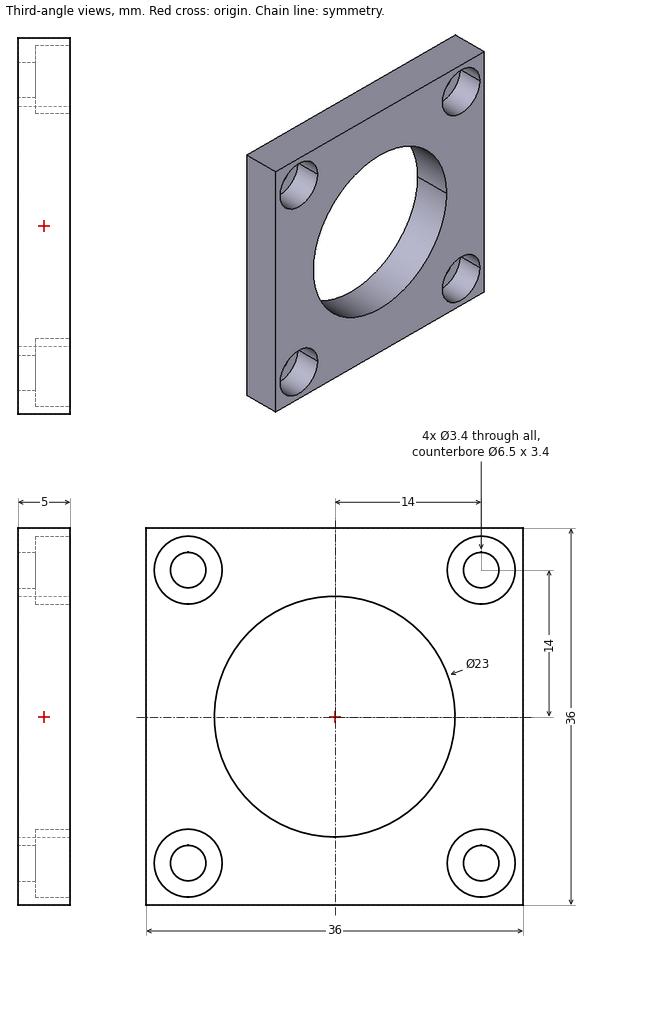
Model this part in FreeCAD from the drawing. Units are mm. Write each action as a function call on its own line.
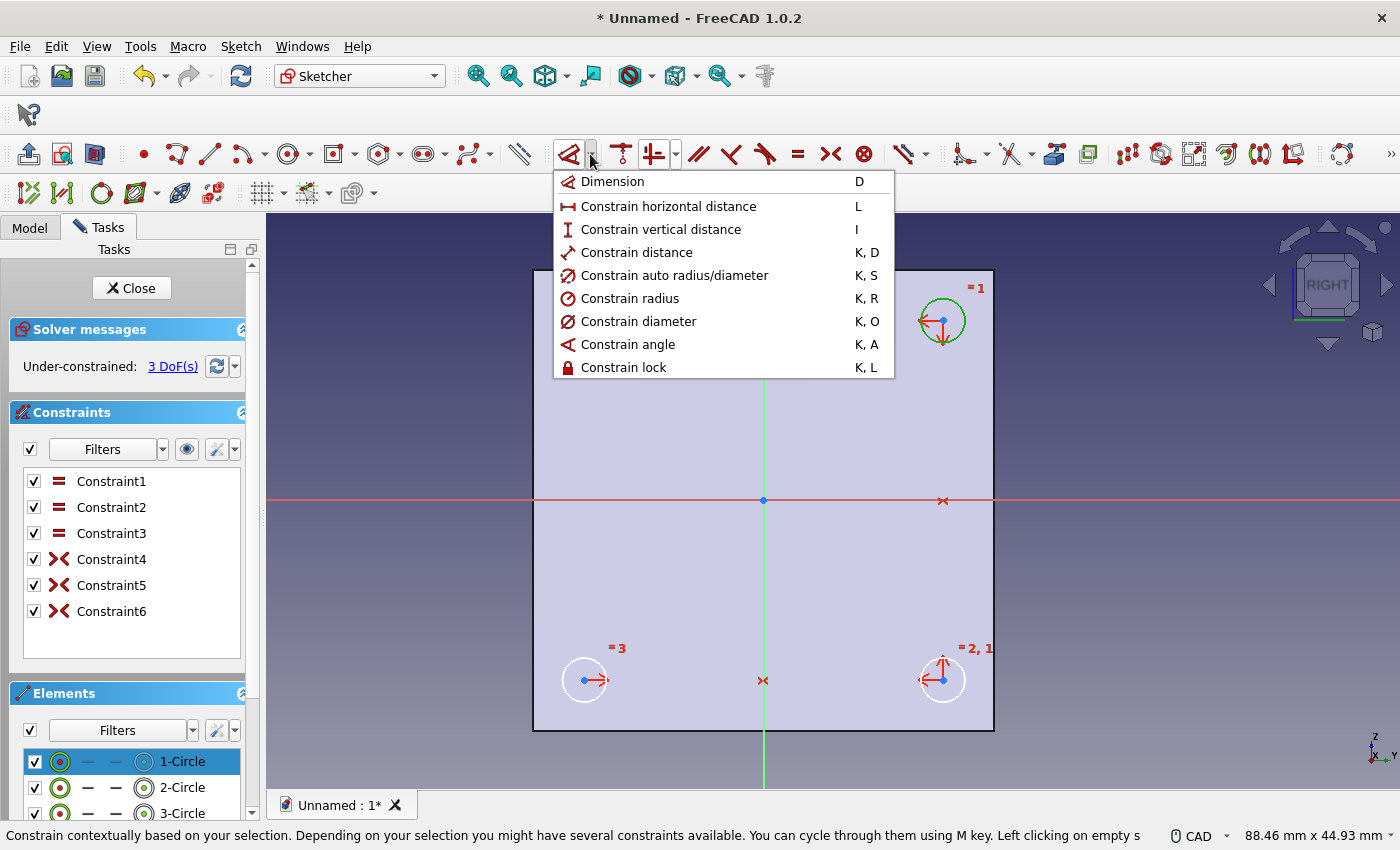
click(724, 322)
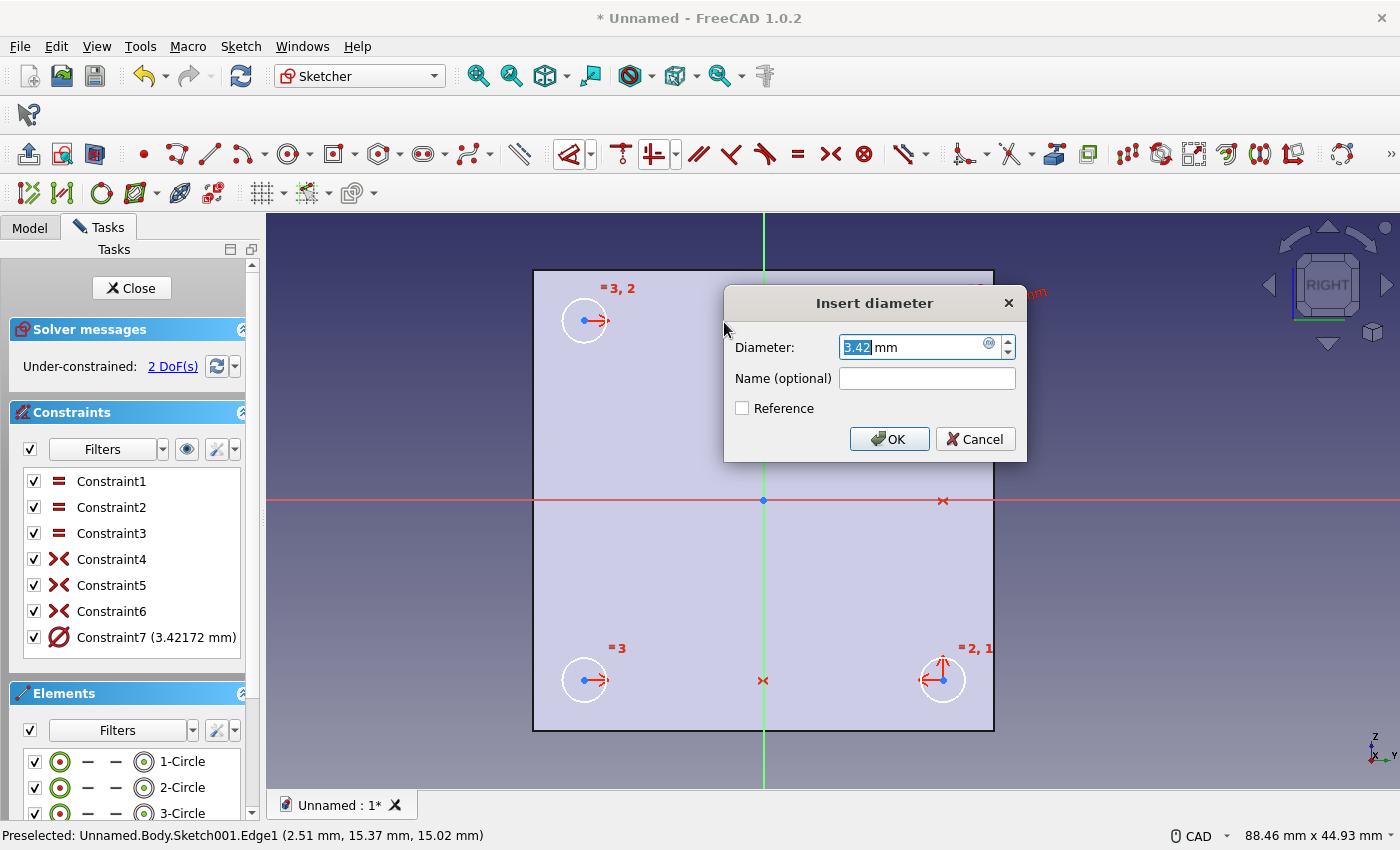
text(3.4)
key(Return)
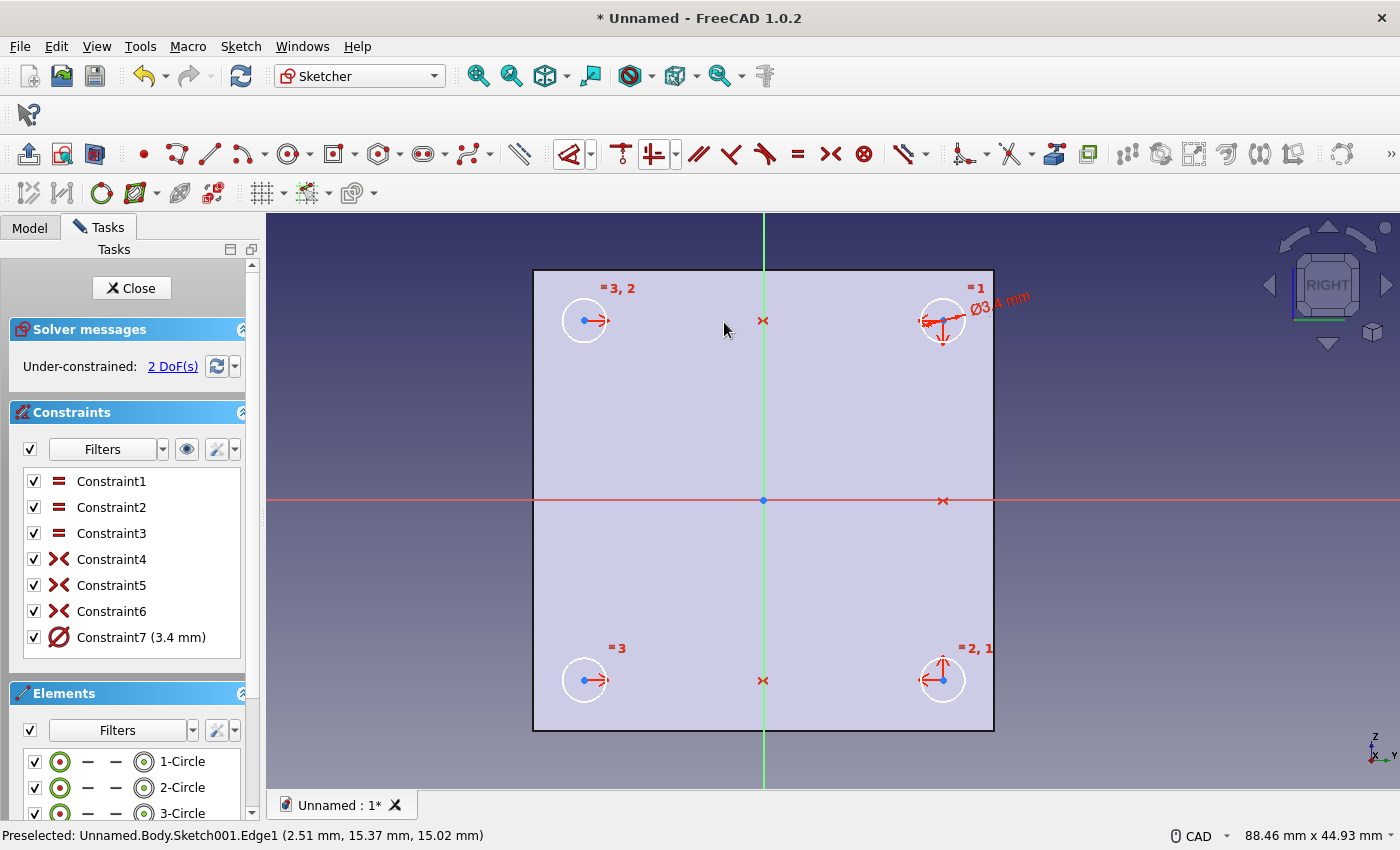
click(943, 321)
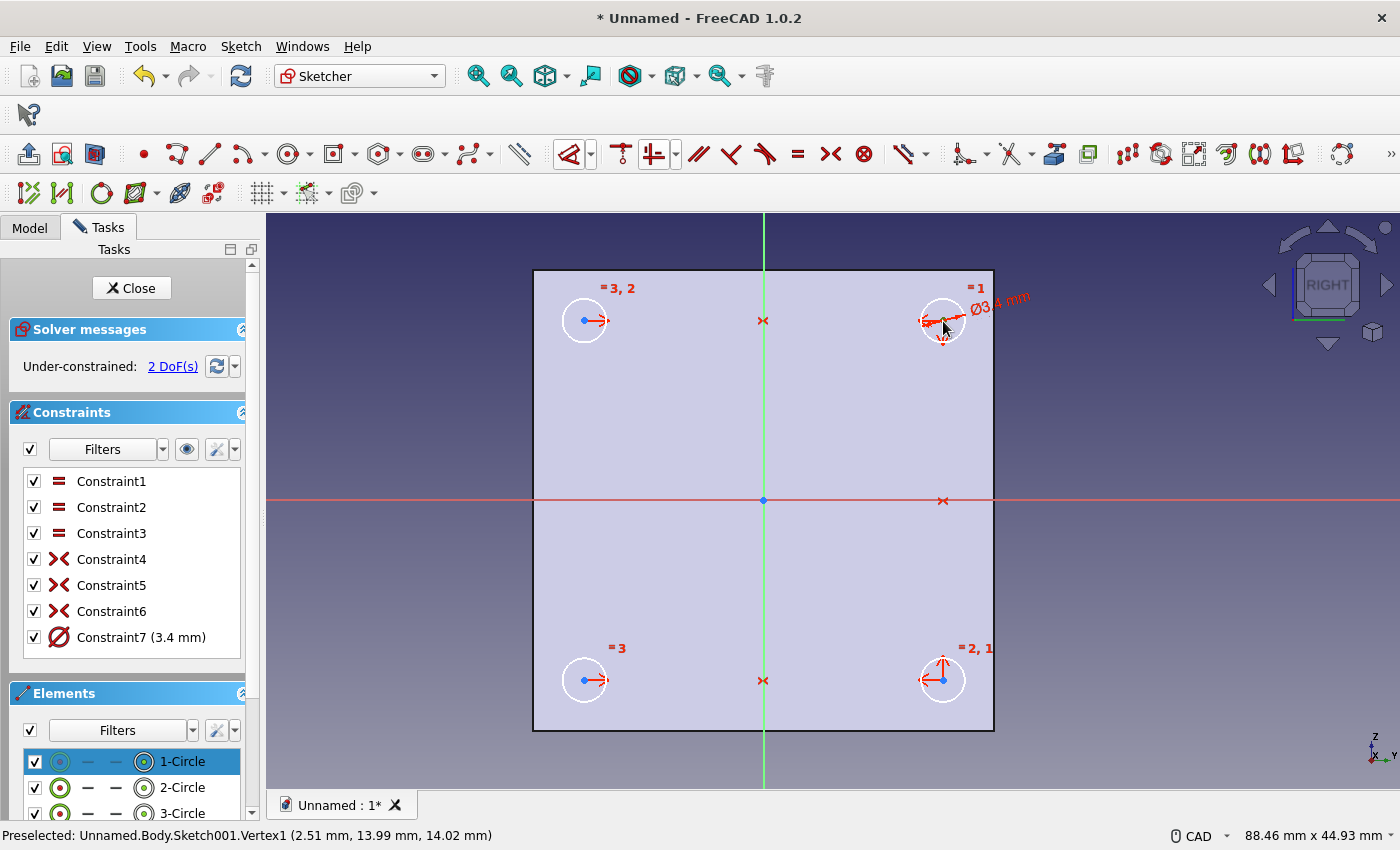
key(l)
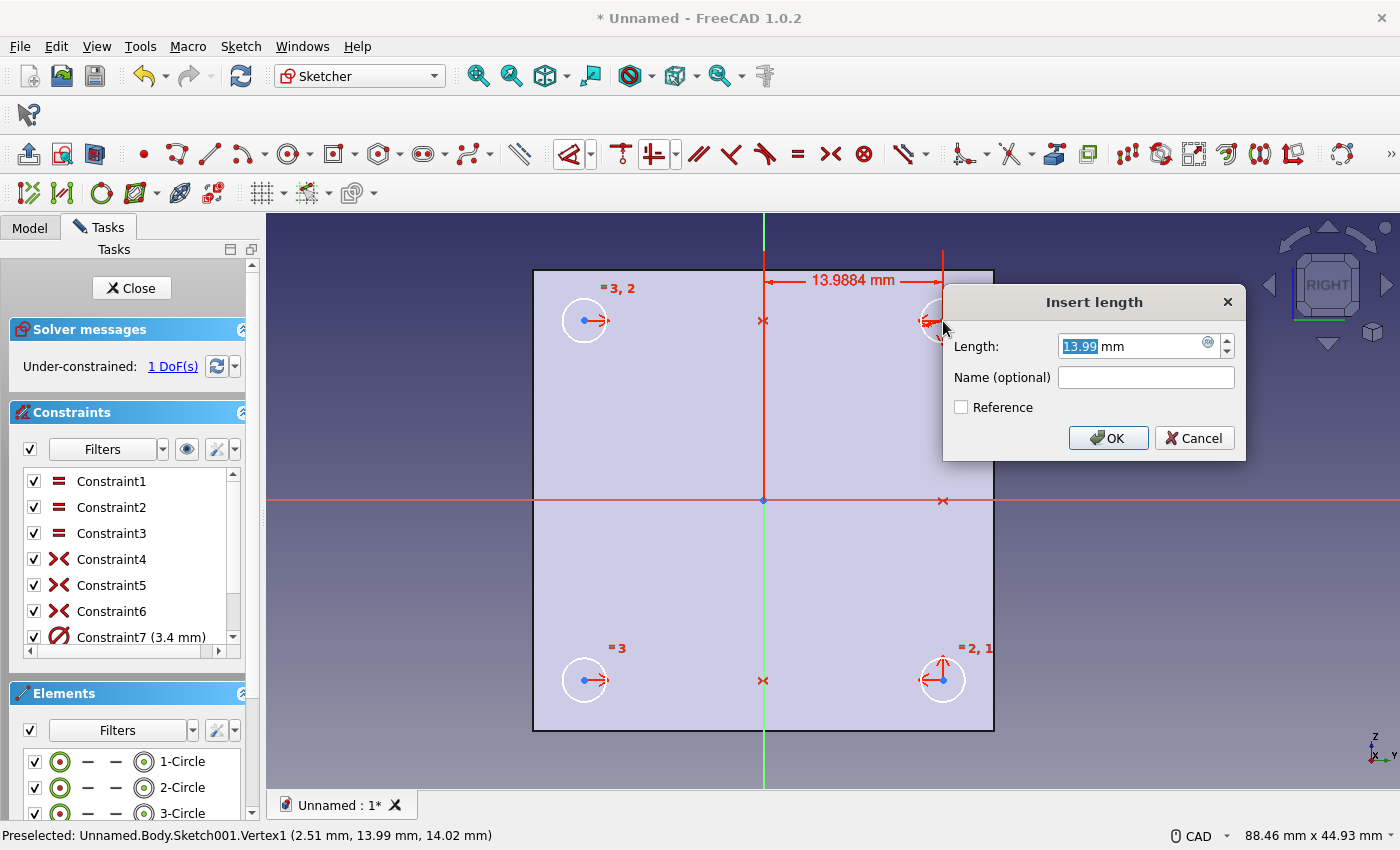
text(14)
key(Return)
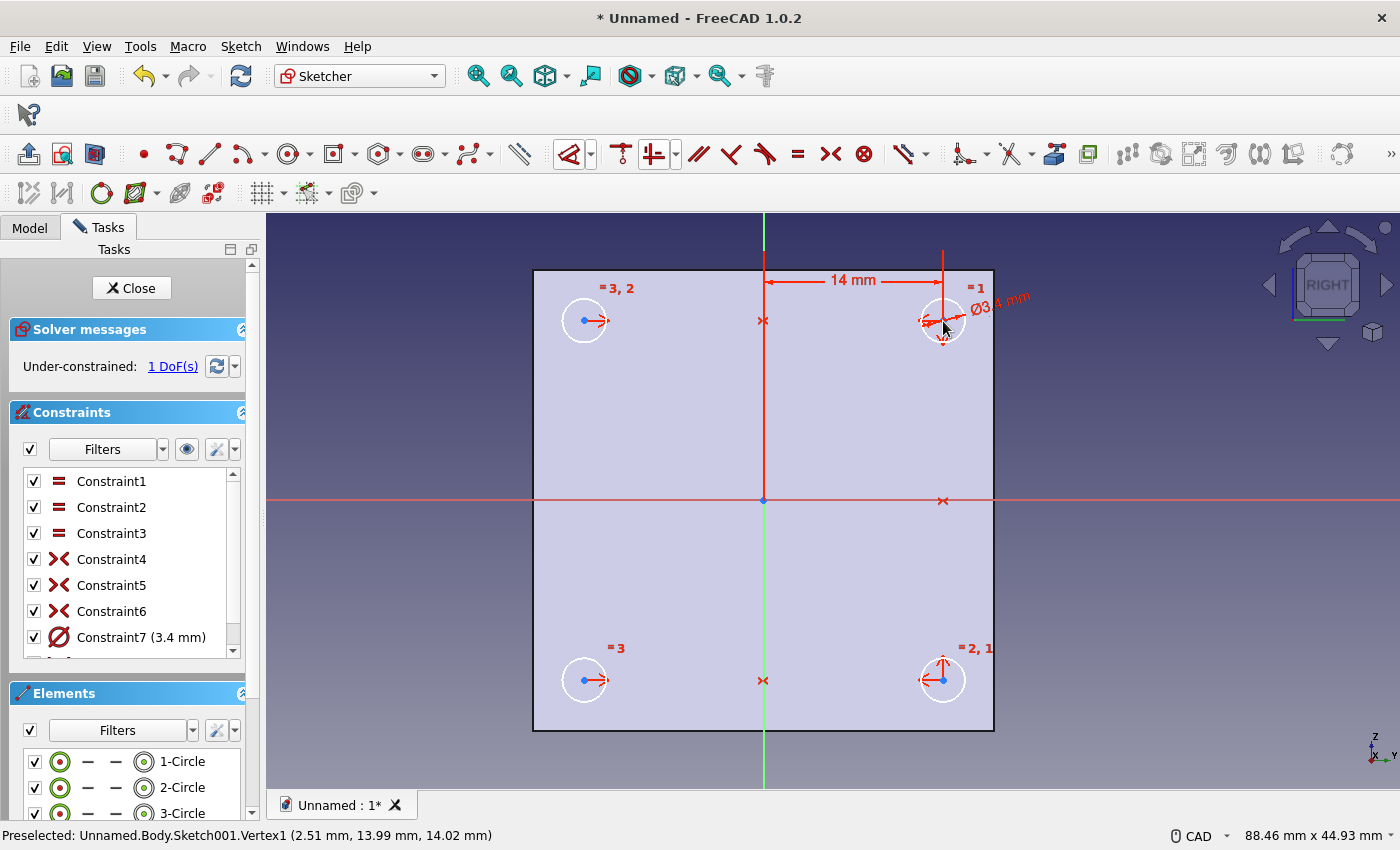
click(943, 321)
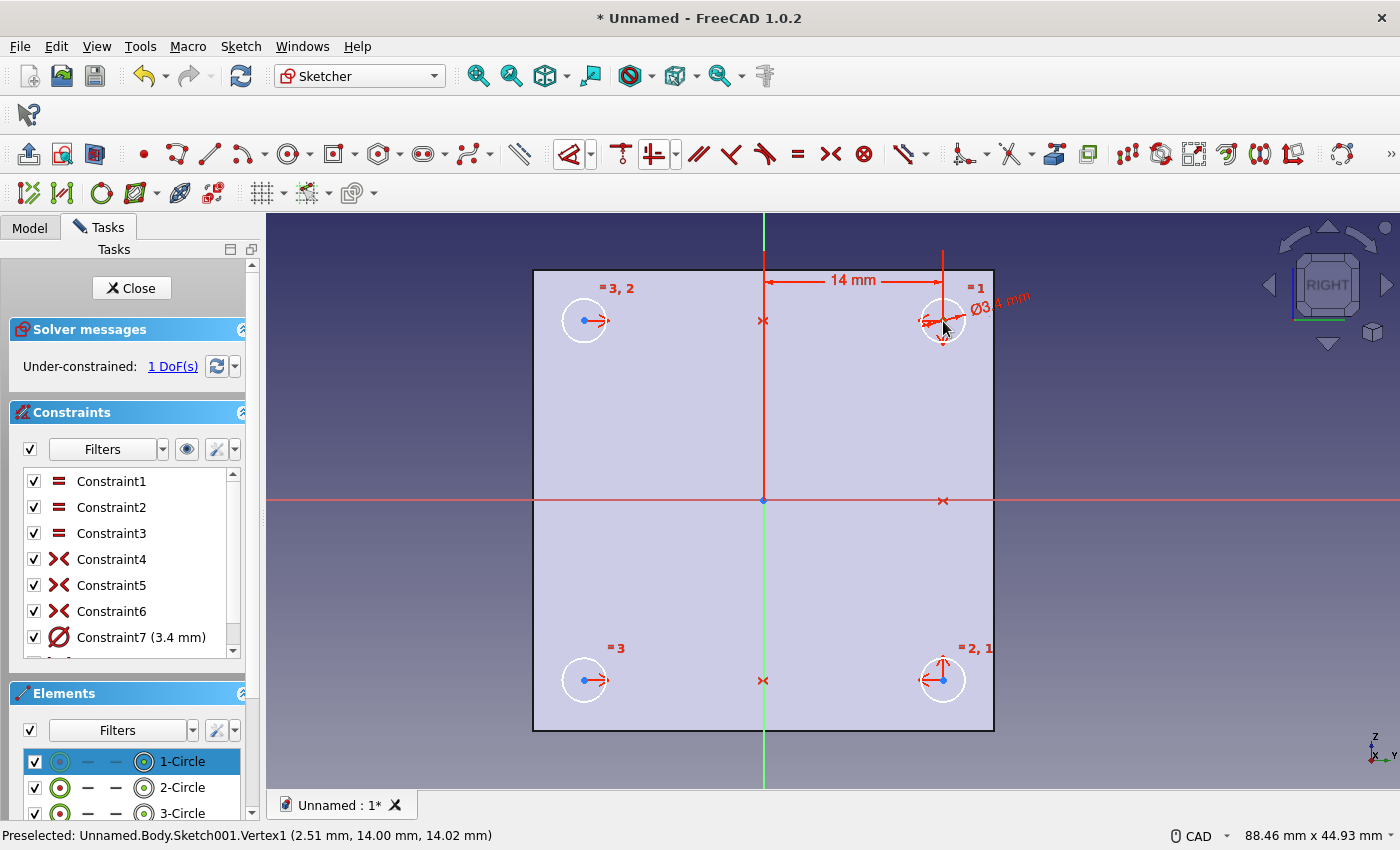
click(590, 154)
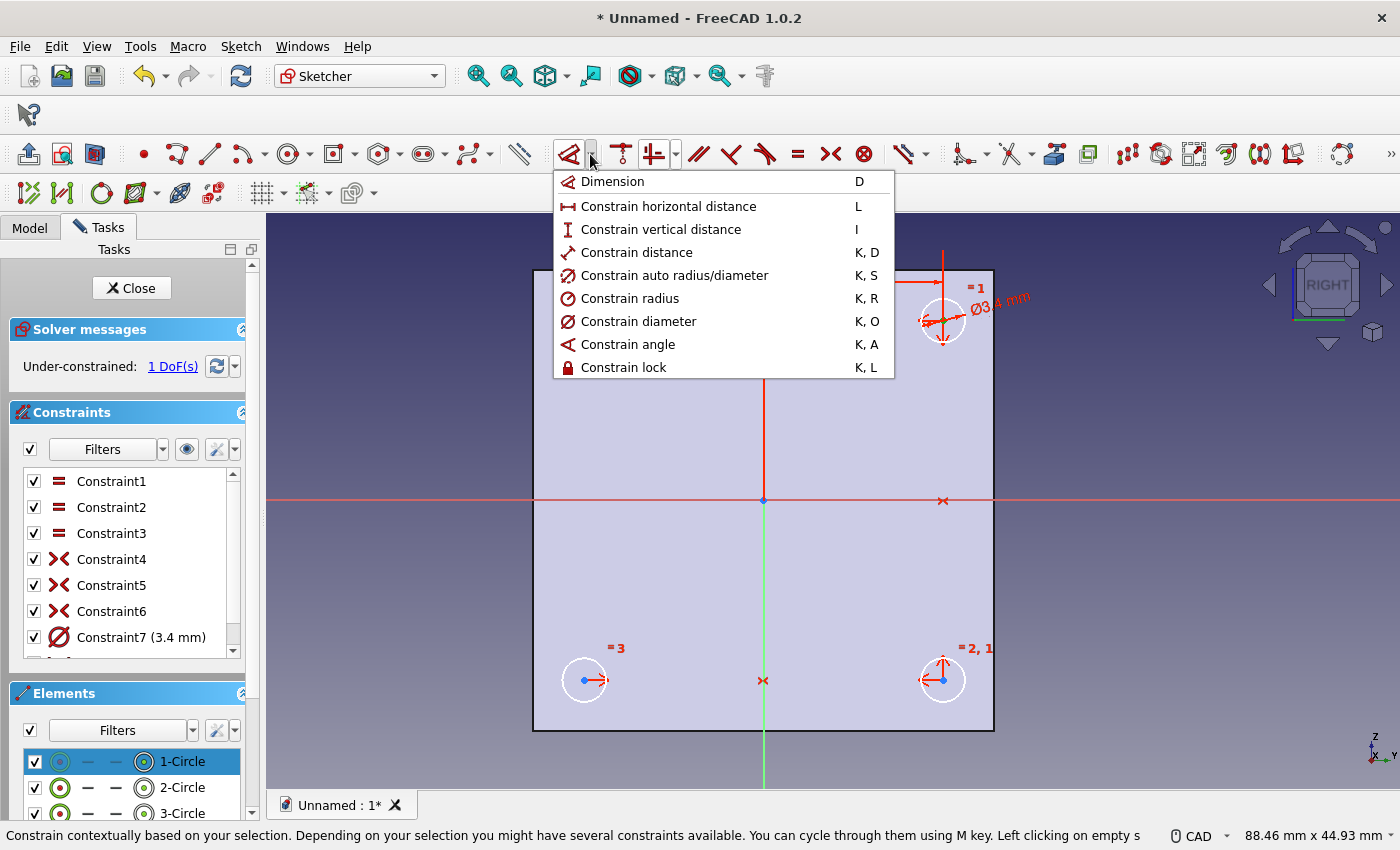
click(724, 230)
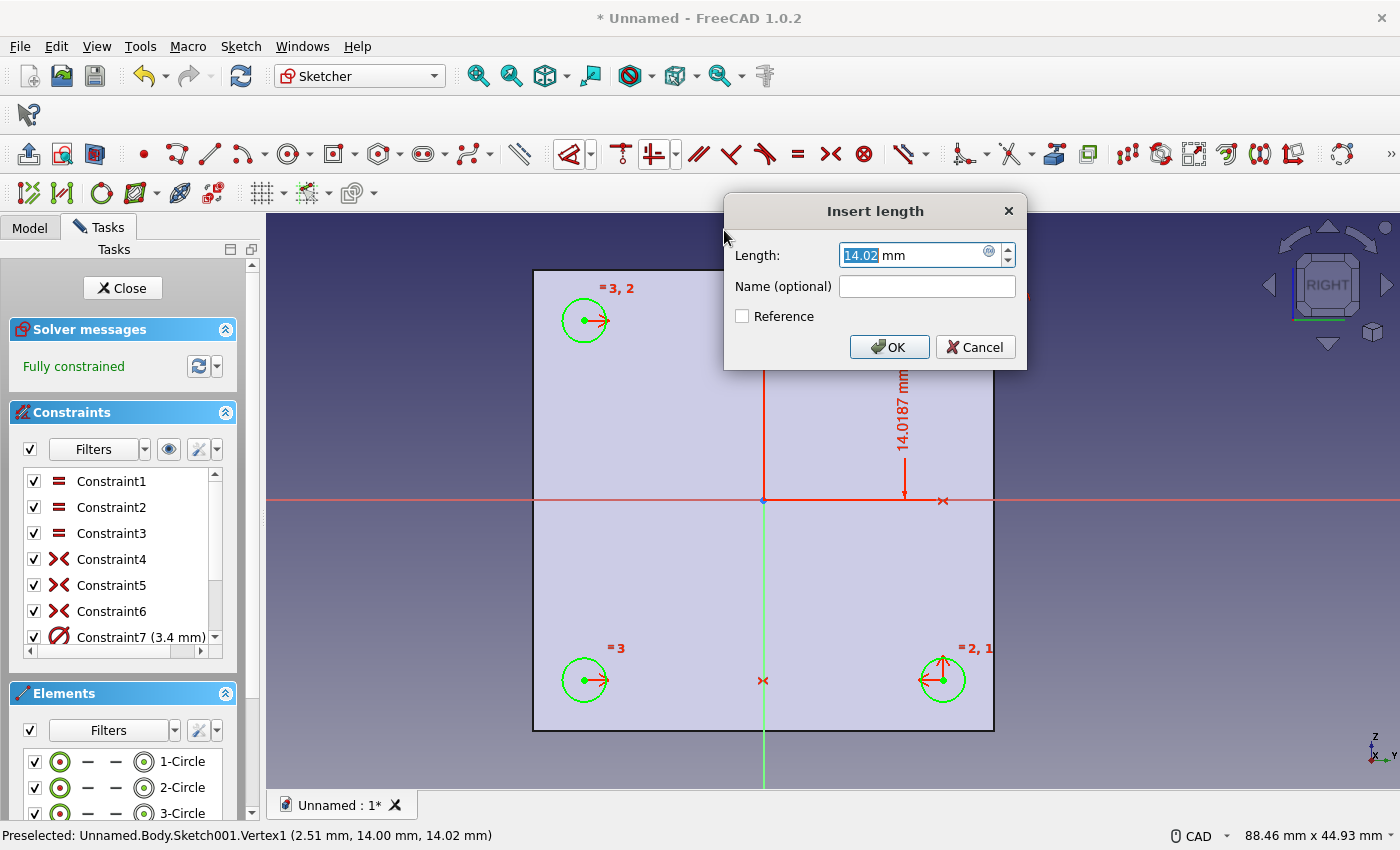
text(14)
key(Return)